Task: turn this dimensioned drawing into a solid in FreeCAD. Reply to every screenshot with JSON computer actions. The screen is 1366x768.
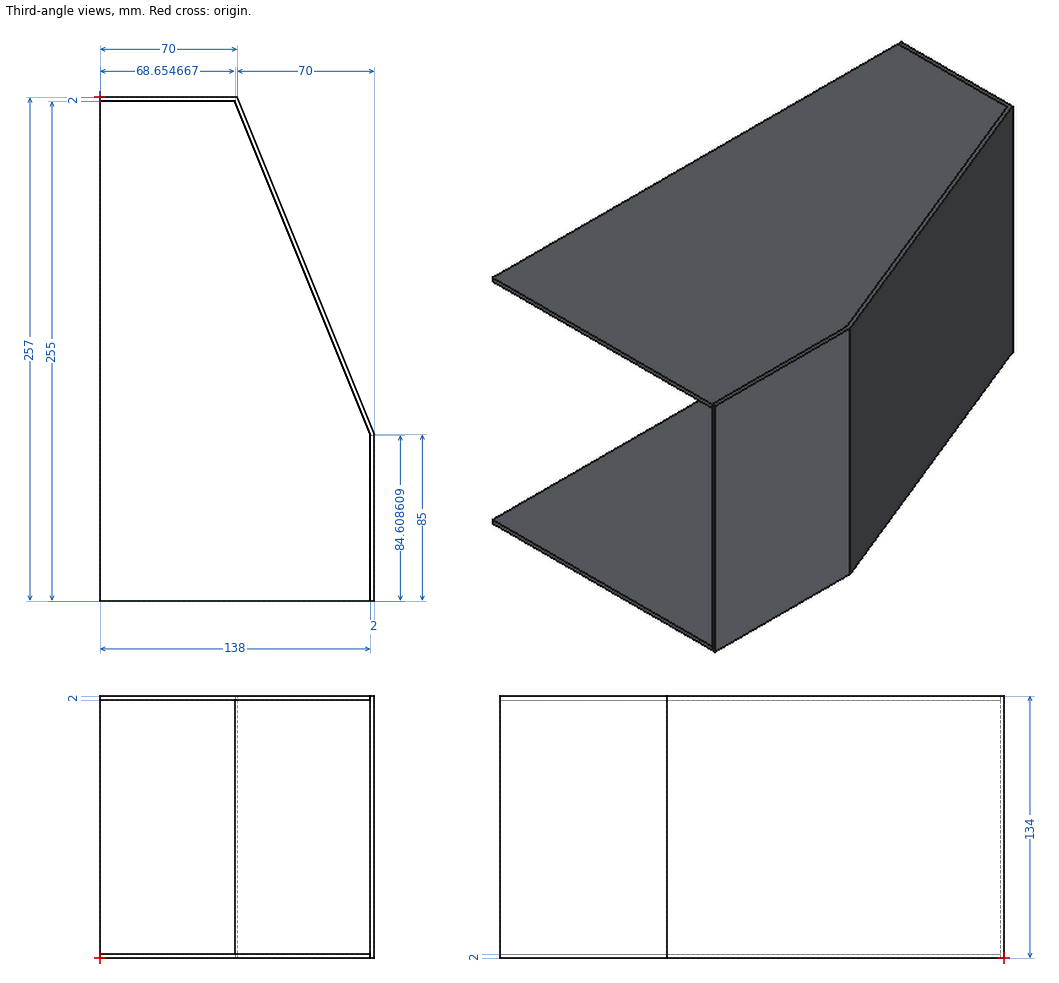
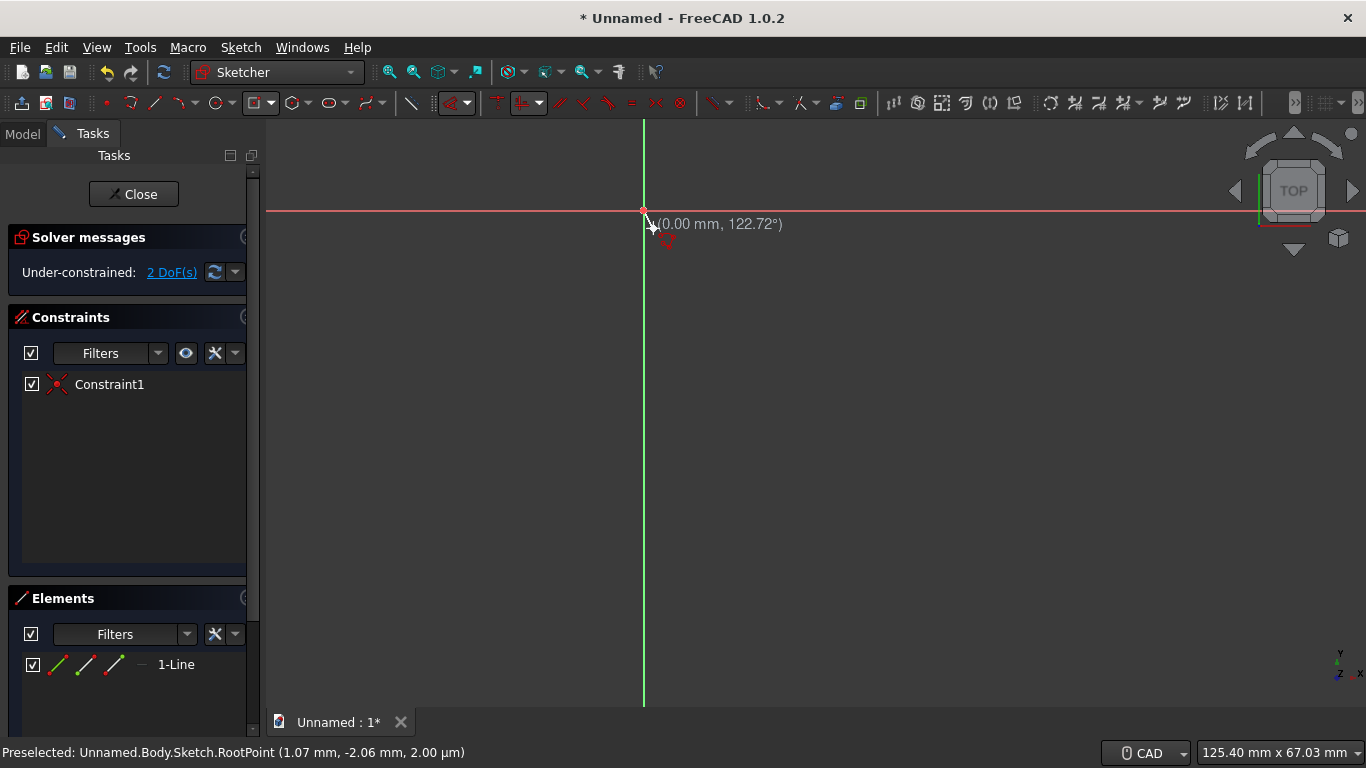
{"action": "scroll", "coordinate": [646, 230], "scroll_direction": "down", "scroll_amount": 9}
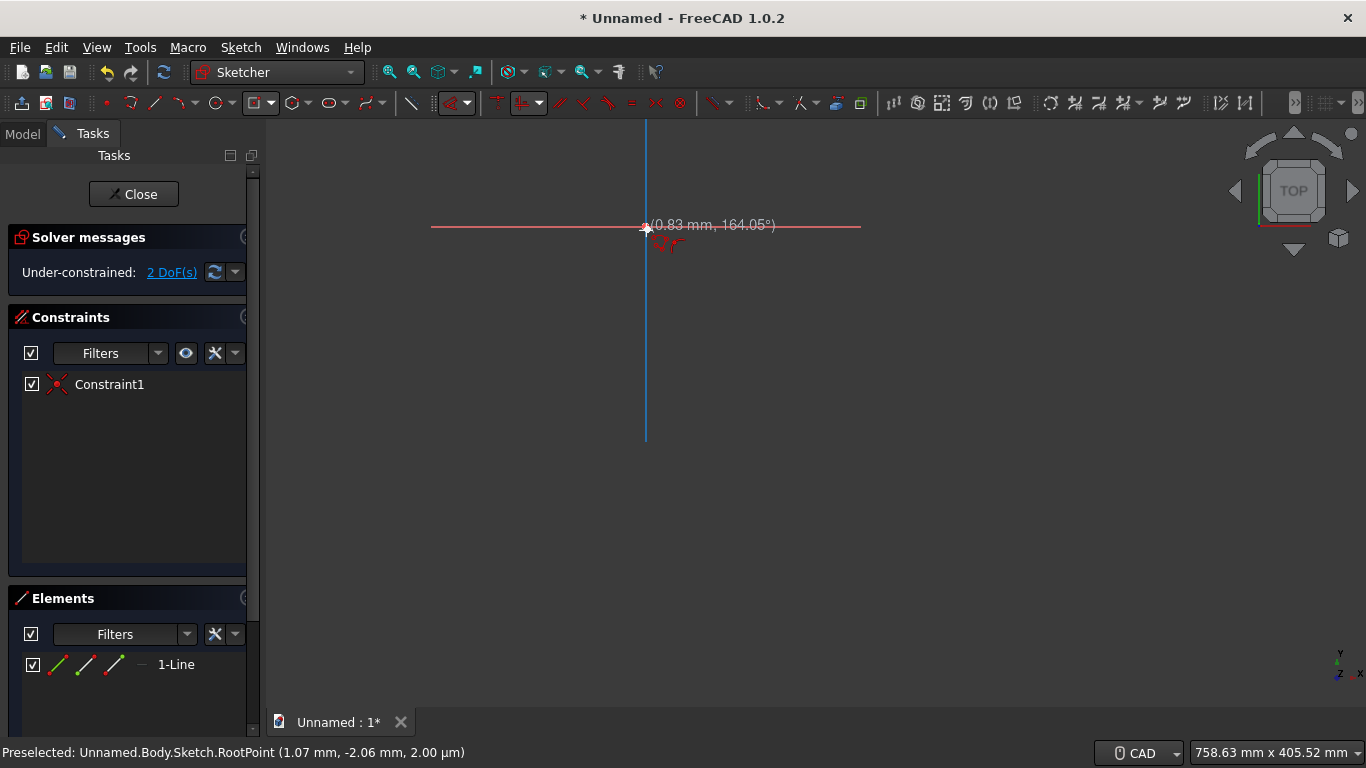
{"action": "scroll", "coordinate": [746, 230], "scroll_direction": "up", "scroll_amount": 9}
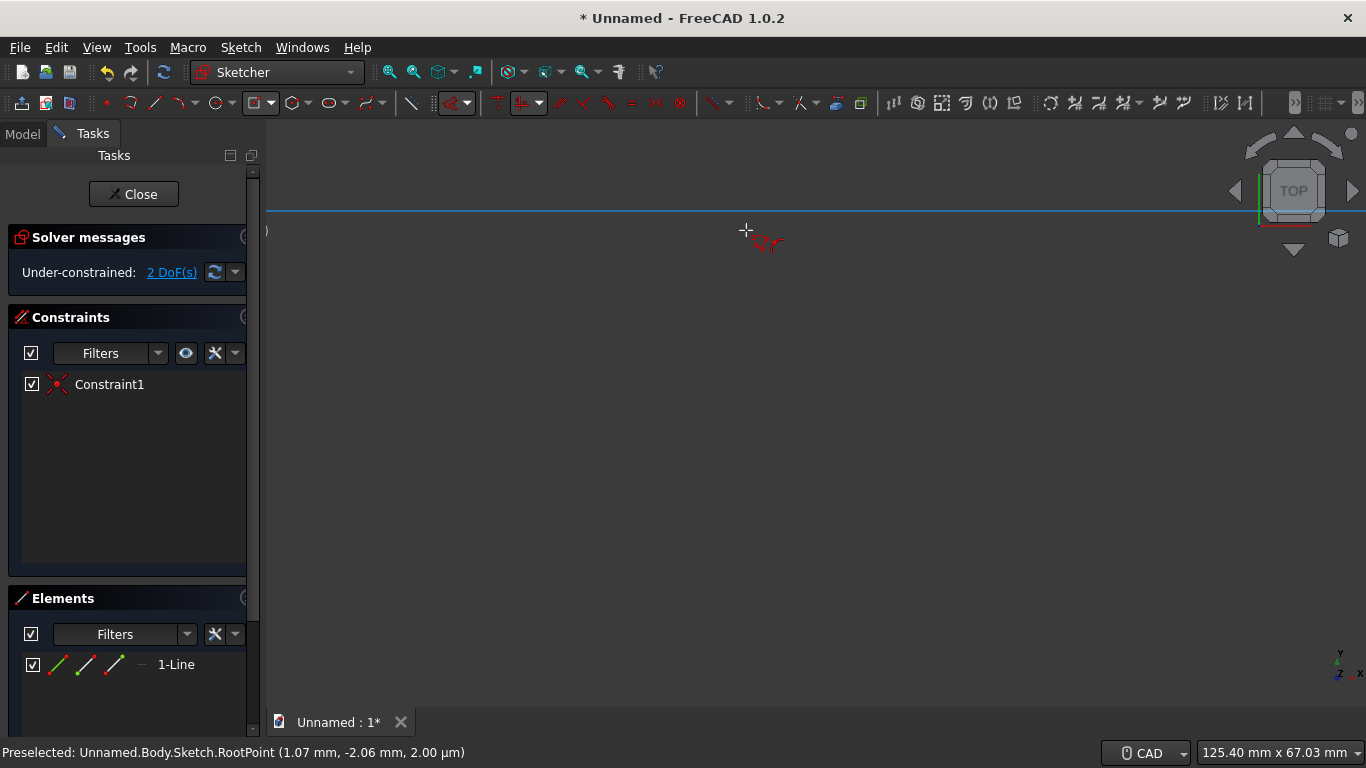
{"action": "left_click", "coordinate": [741, 228]}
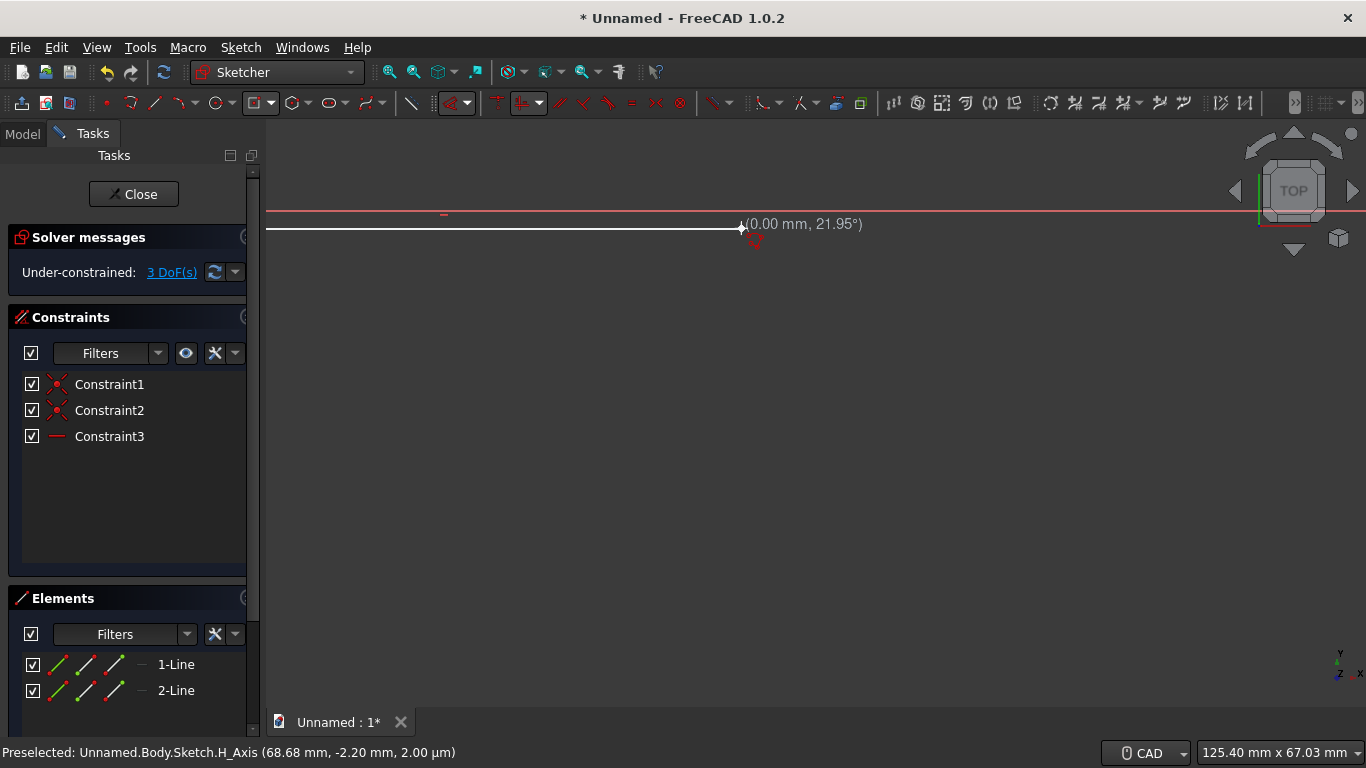
{"action": "scroll", "coordinate": [746, 230], "scroll_direction": "down", "scroll_amount": 9}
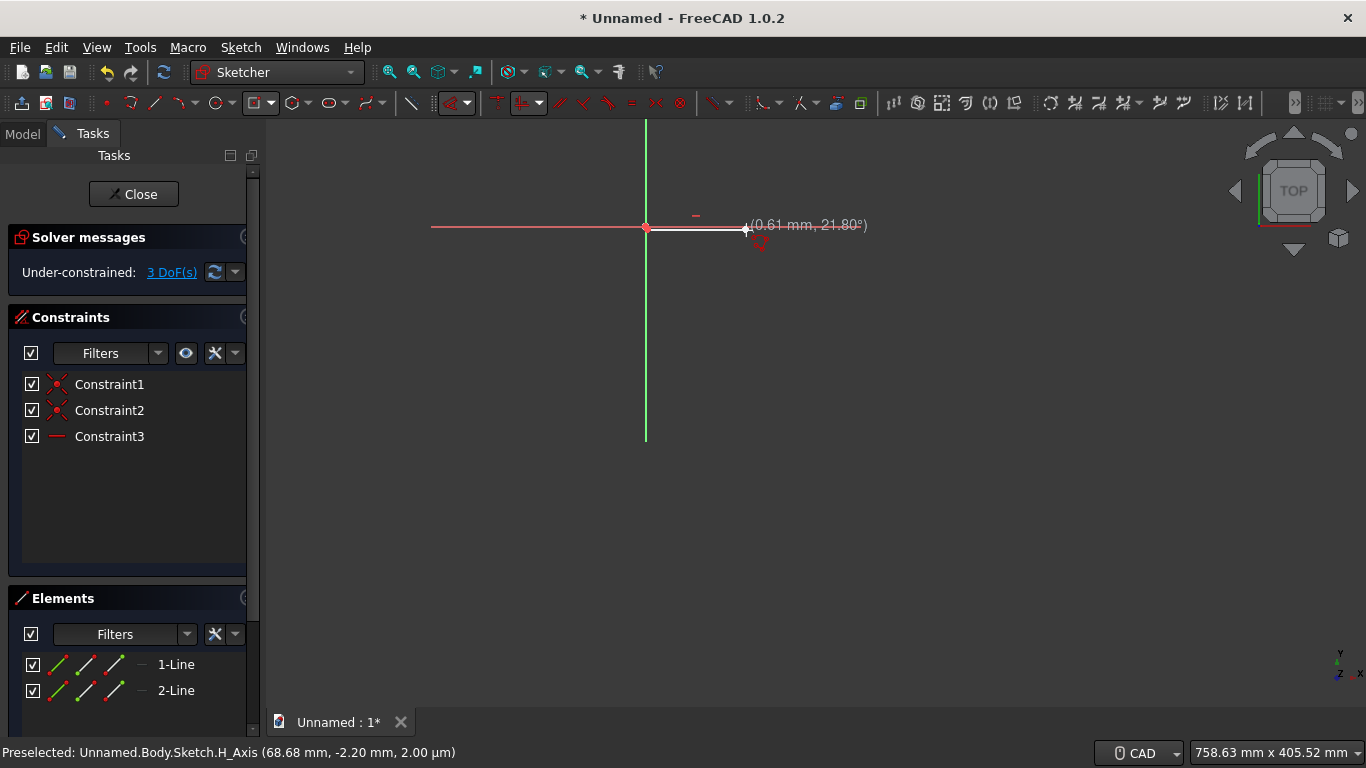
{"action": "left_click", "coordinate": [846, 477]}
{"action": "left_click", "coordinate": [846, 600]}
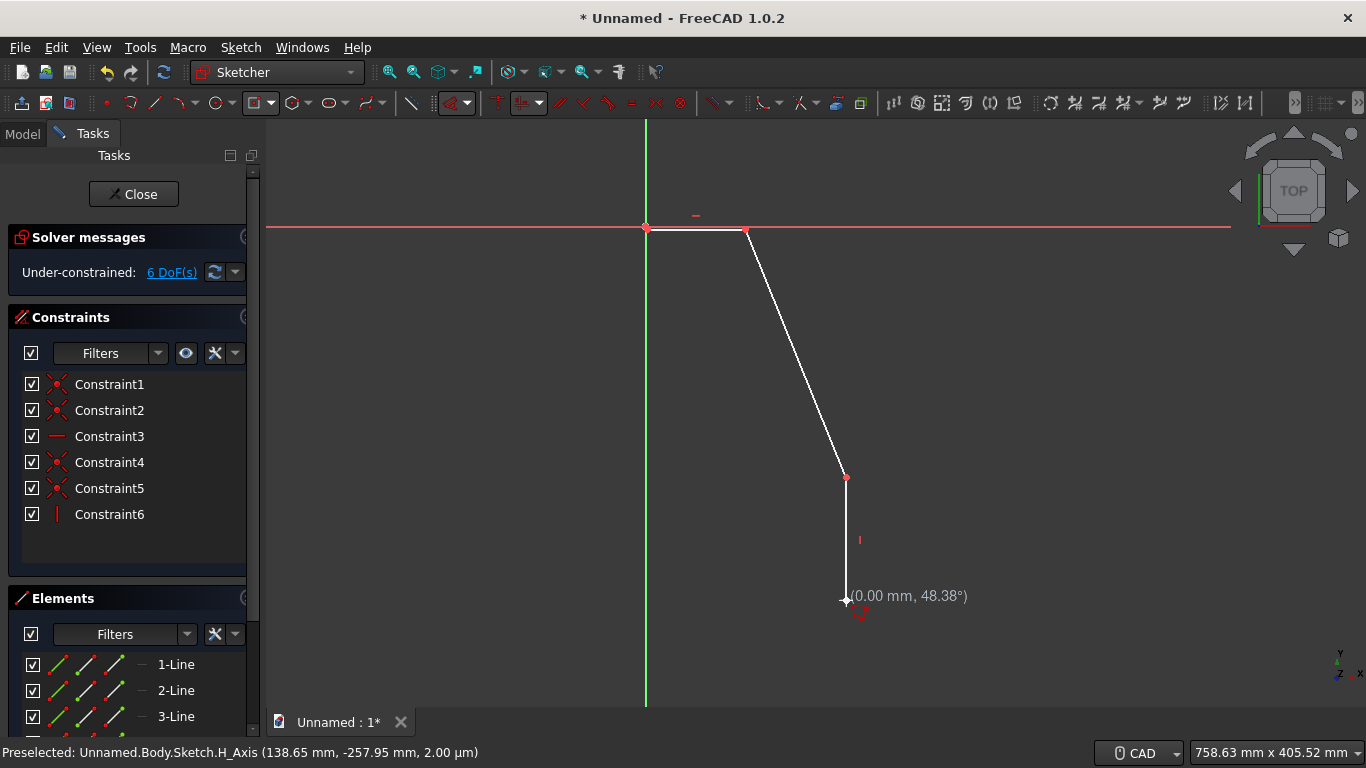
{"action": "scroll", "coordinate": [849, 600], "scroll_direction": "up", "scroll_amount": 9}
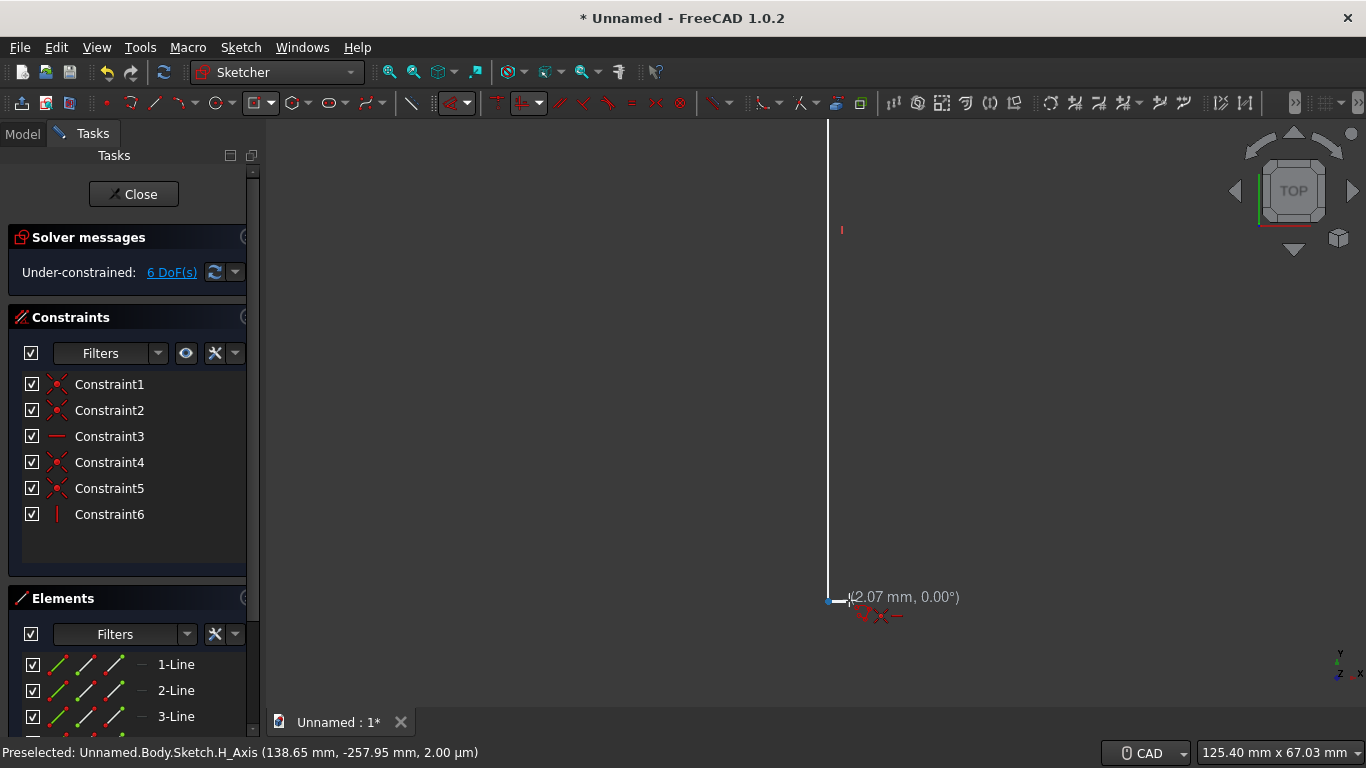
{"action": "left_click", "coordinate": [846, 596]}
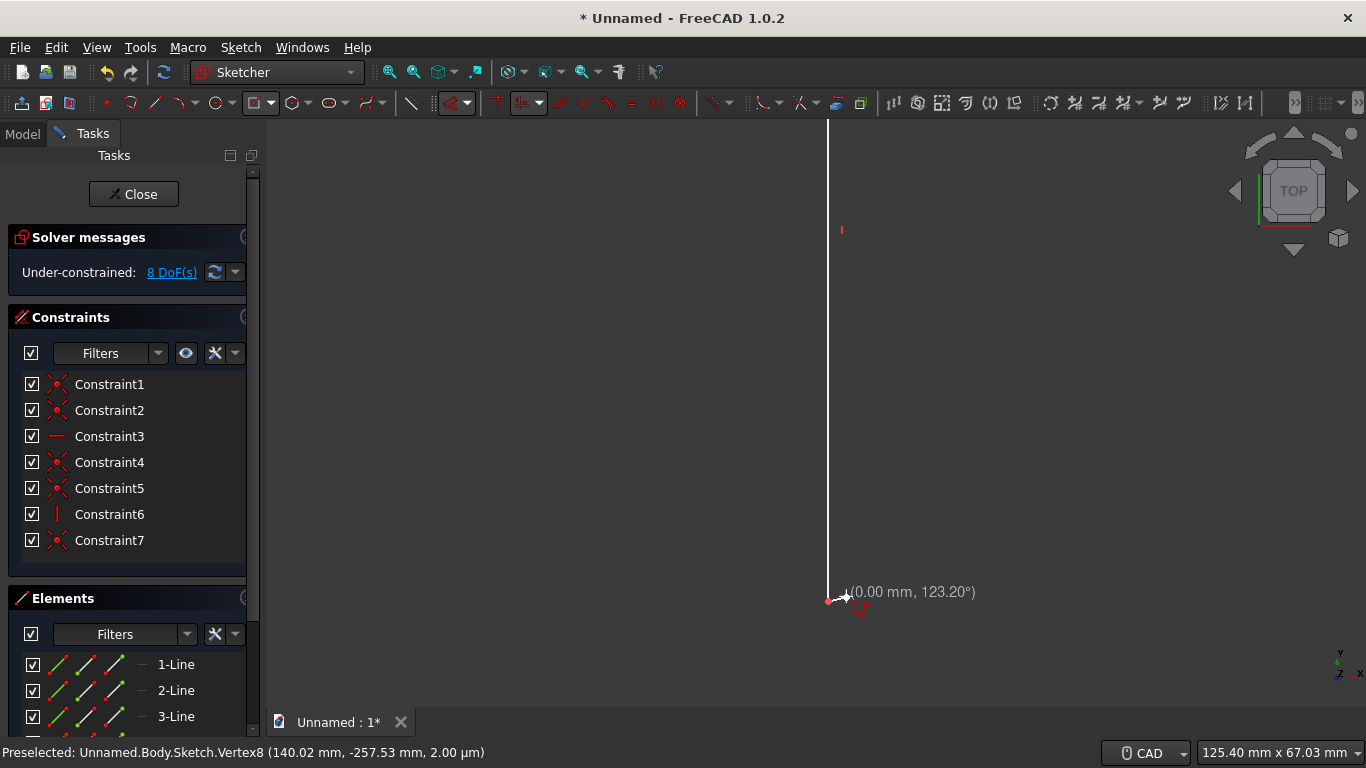
{"action": "scroll", "coordinate": [850, 600], "scroll_direction": "down", "scroll_amount": 9}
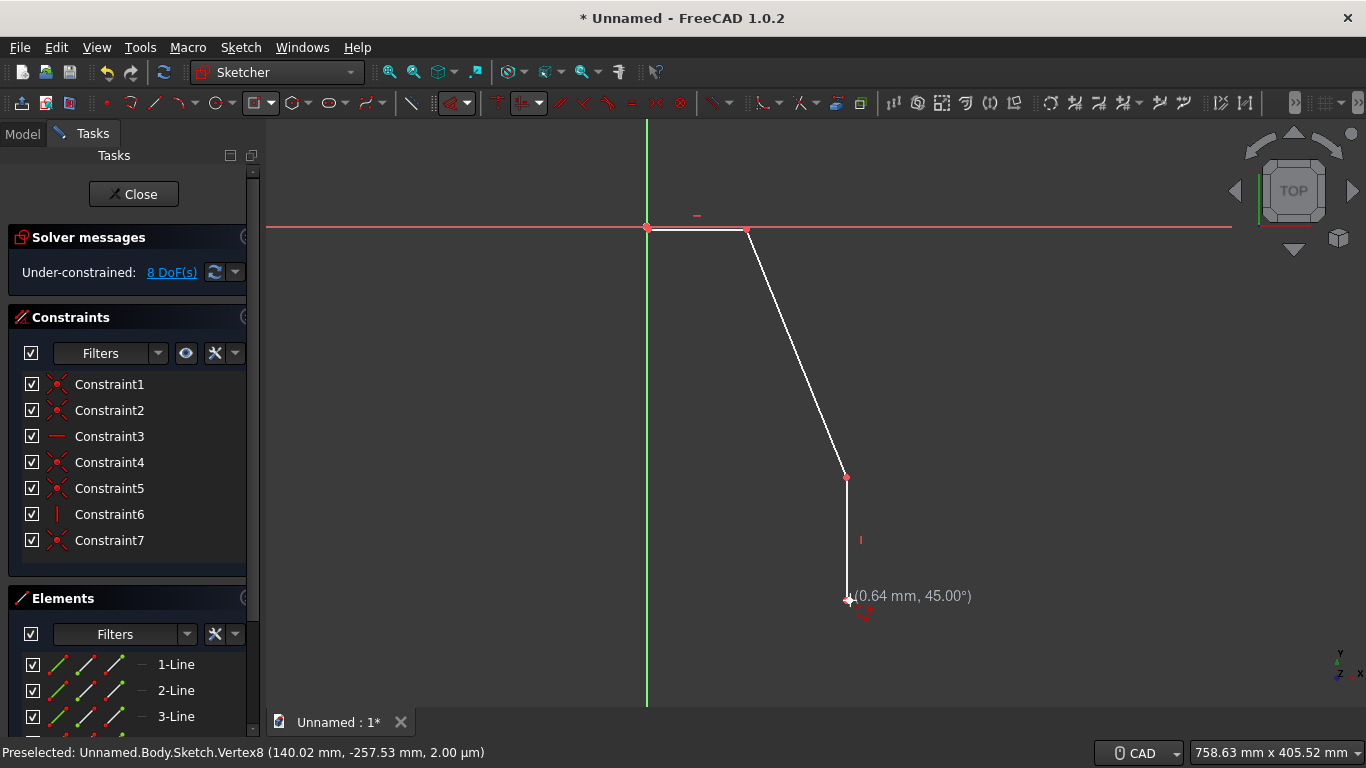
{"action": "scroll", "coordinate": [850, 476], "scroll_direction": "up", "scroll_amount": 9}